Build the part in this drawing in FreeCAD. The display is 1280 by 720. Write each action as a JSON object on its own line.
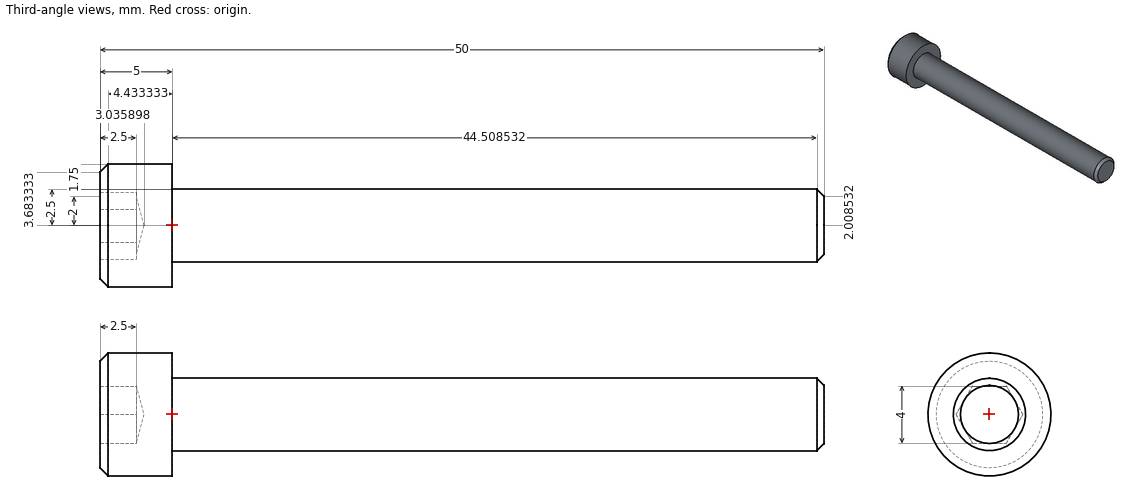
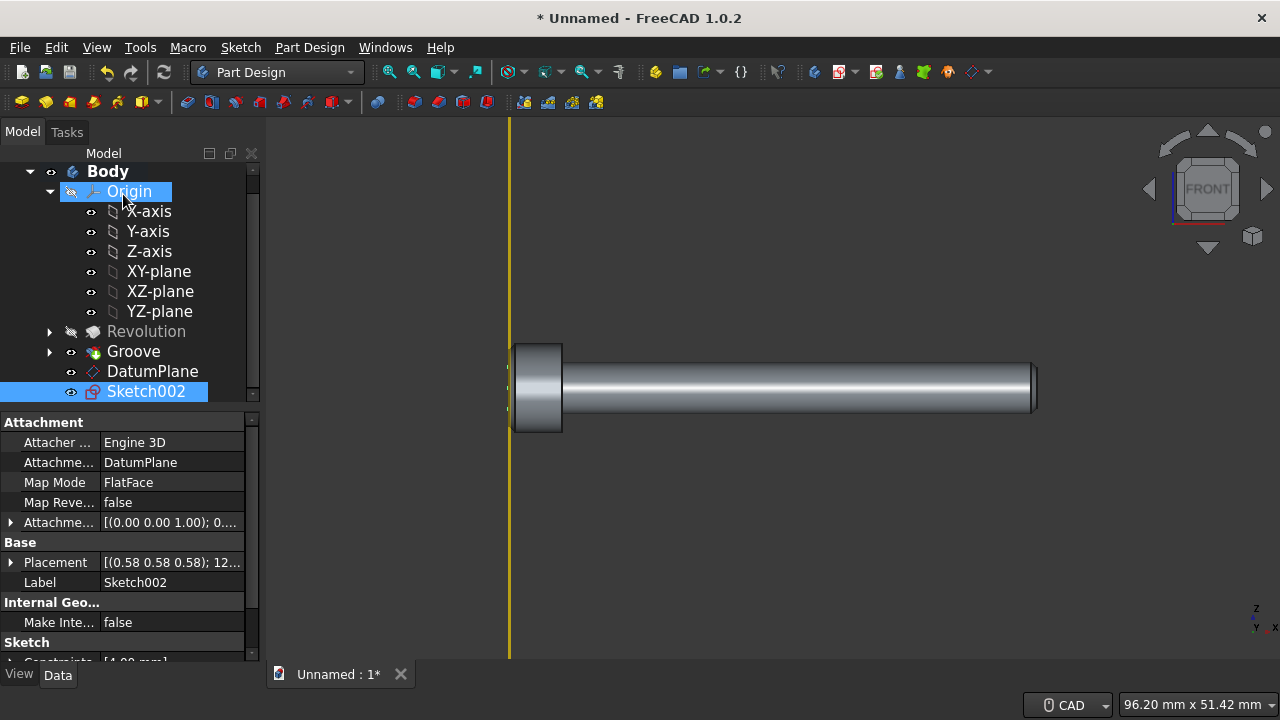
{"action": "left_click", "coordinate": [188, 102]}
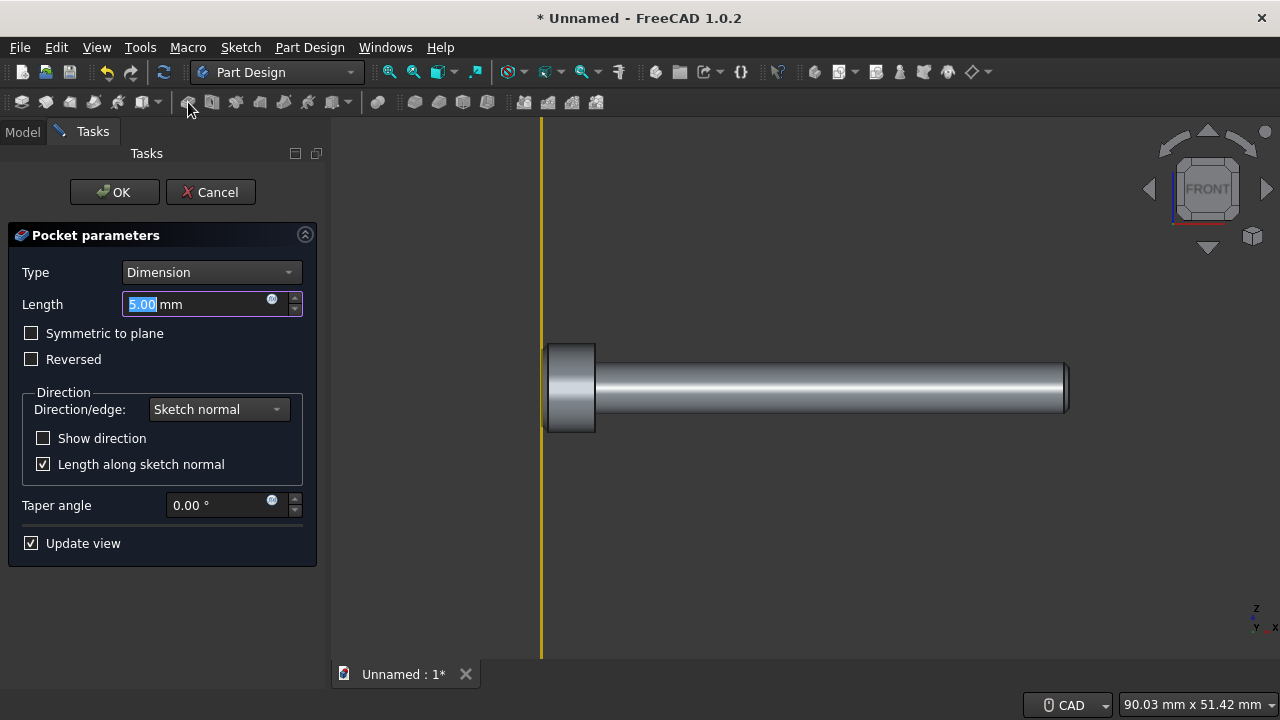
{"action": "type", "text": "2.5"}
{"action": "key", "text": "Tab"}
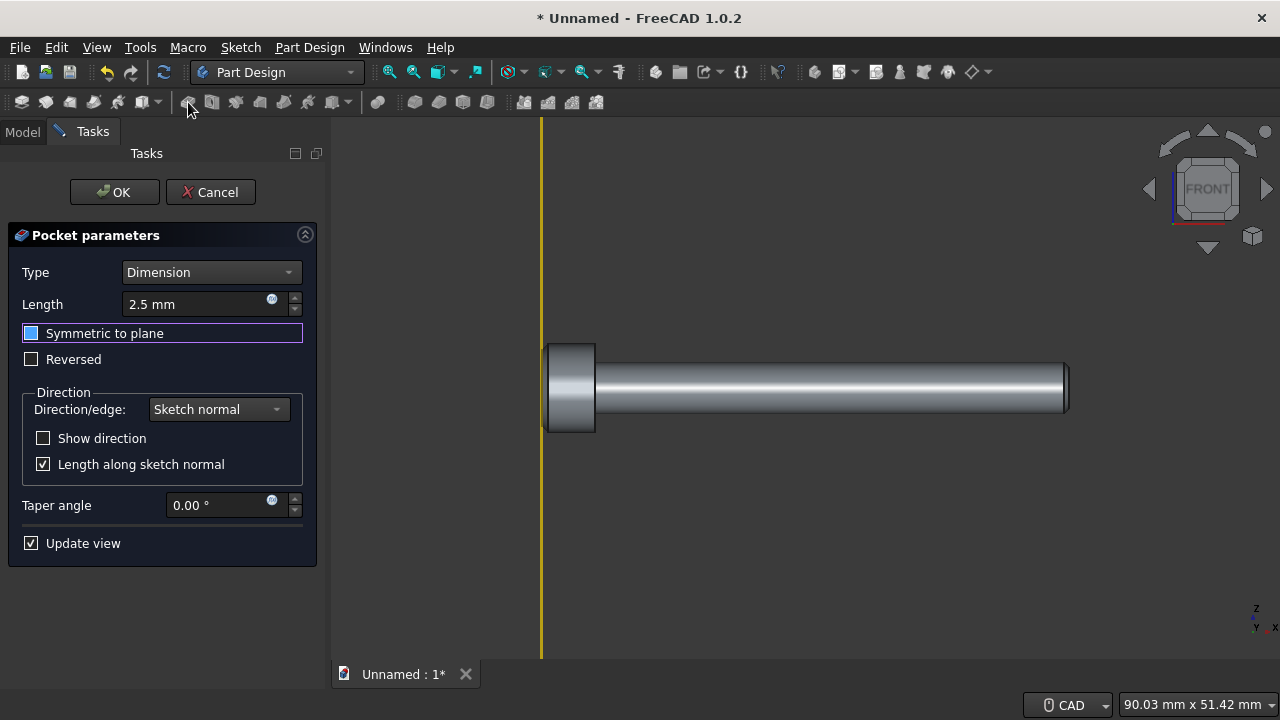
{"action": "left_click", "coordinate": [30, 359]}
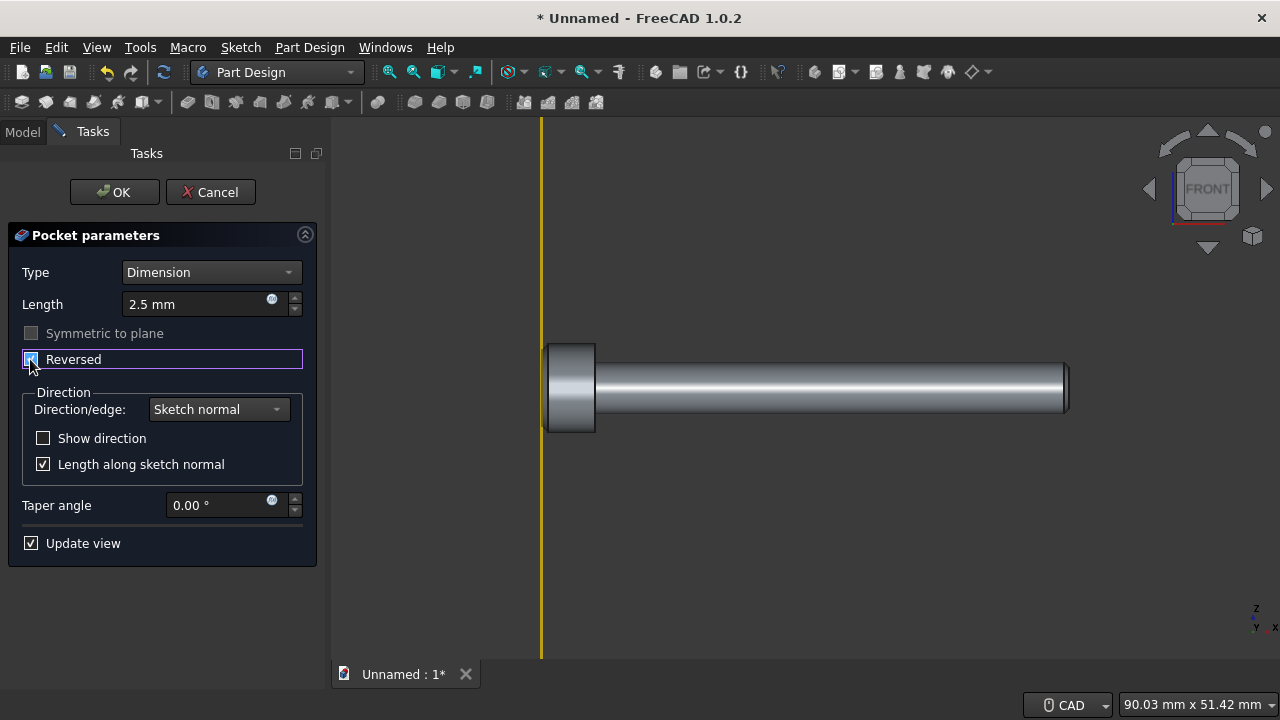
{"action": "left_click", "coordinate": [115, 192]}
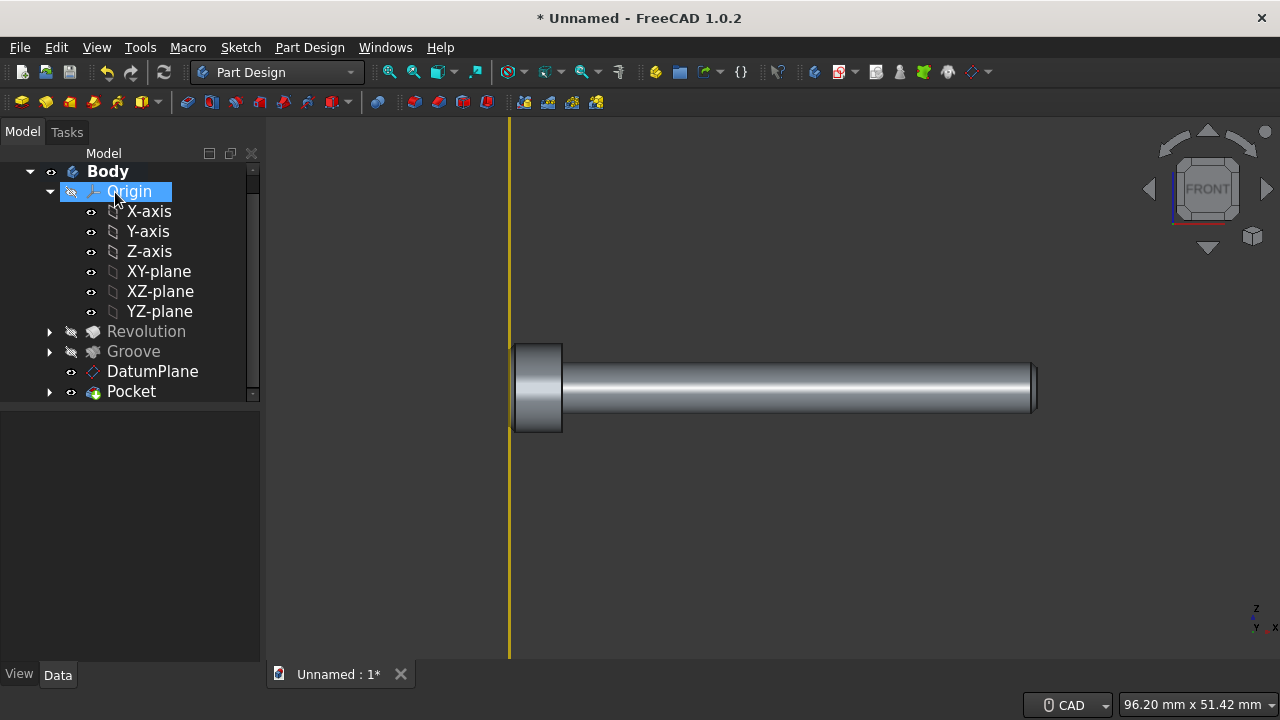
{"action": "left_click", "coordinate": [116, 372]}
{"action": "key", "text": "space"}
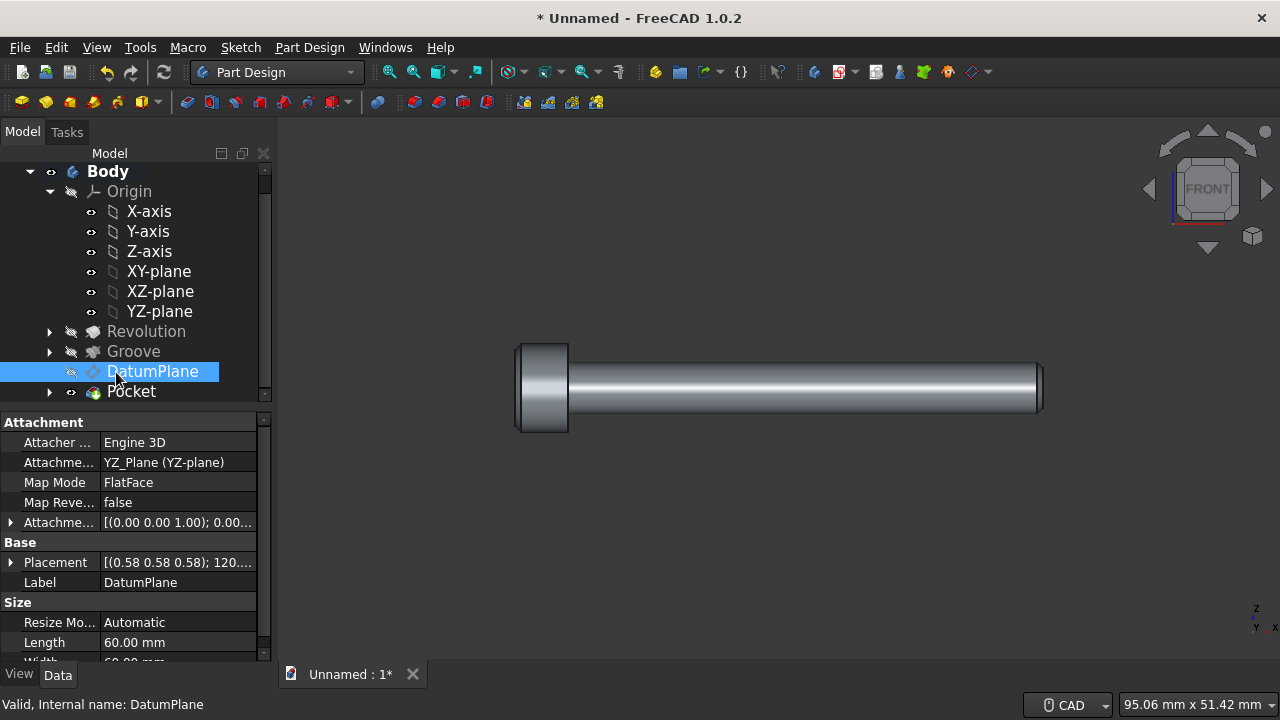
{"action": "key", "text": "0"}